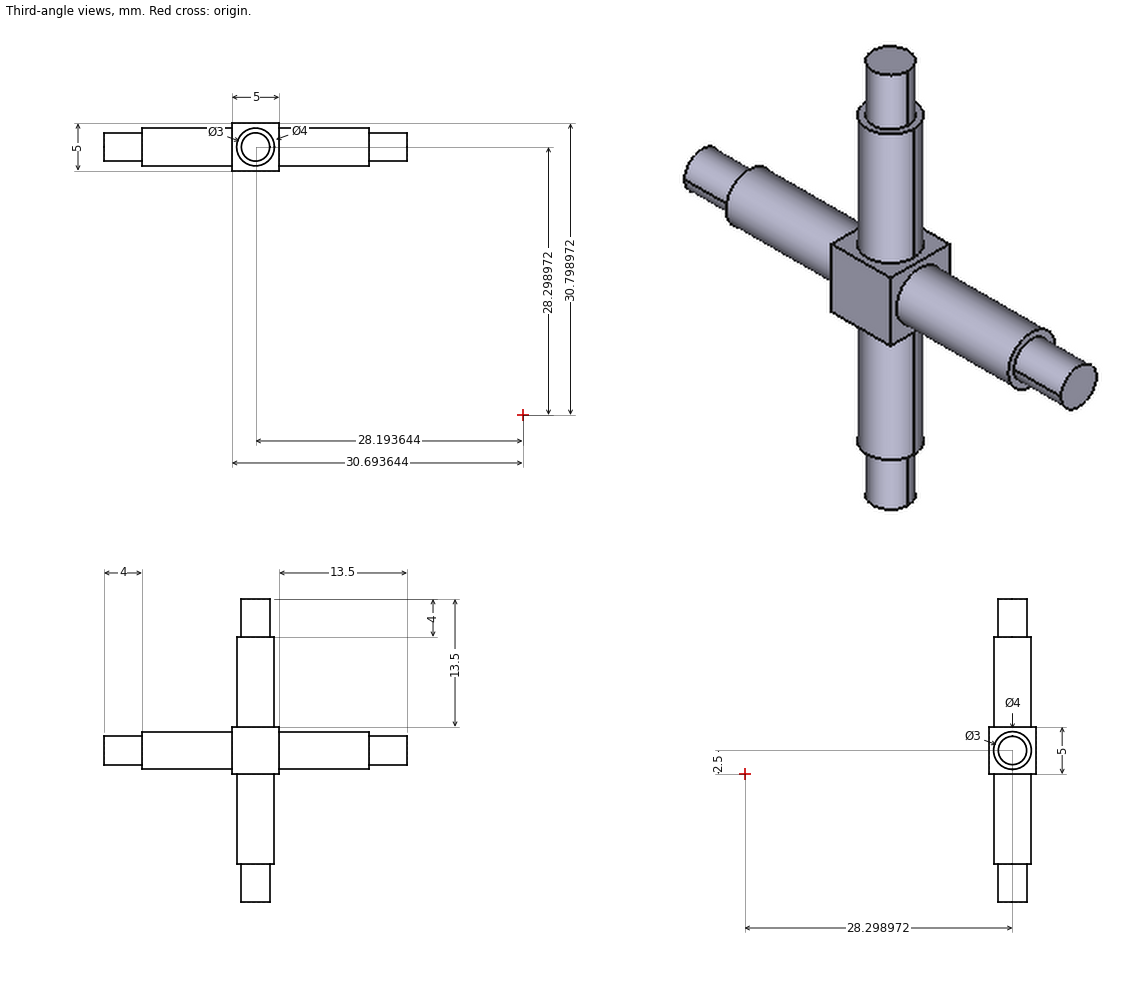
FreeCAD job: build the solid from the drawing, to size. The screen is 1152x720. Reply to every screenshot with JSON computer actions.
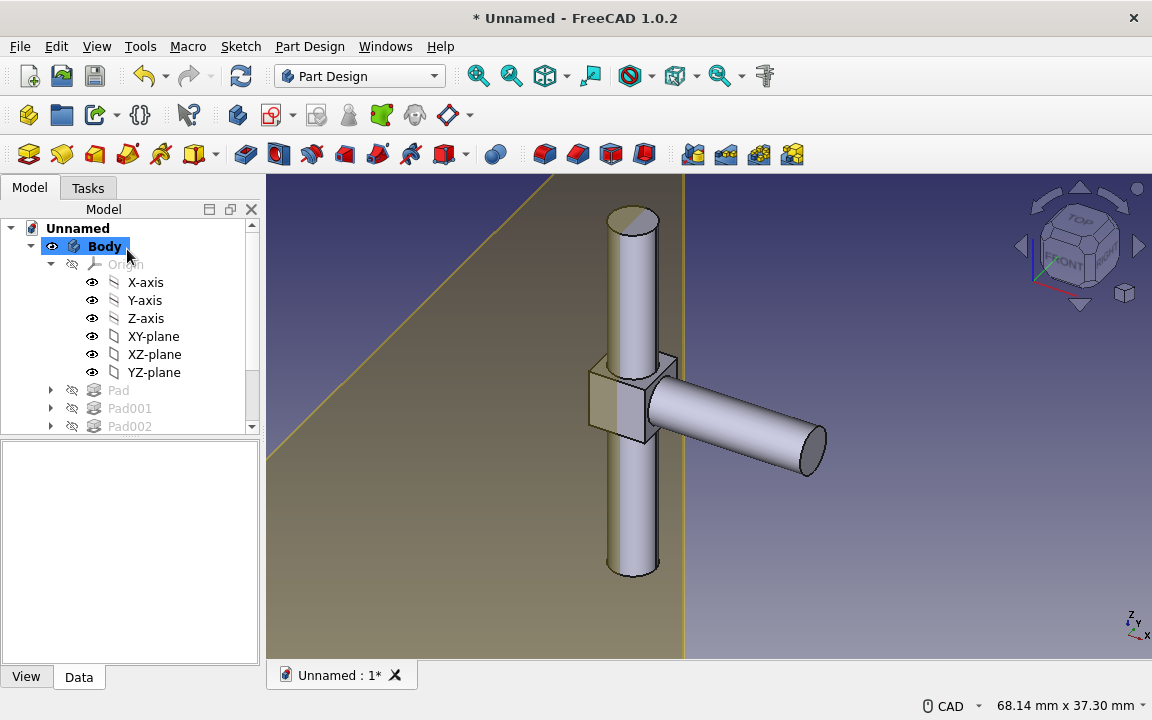
{"action": "left_click", "coordinate": [117, 426]}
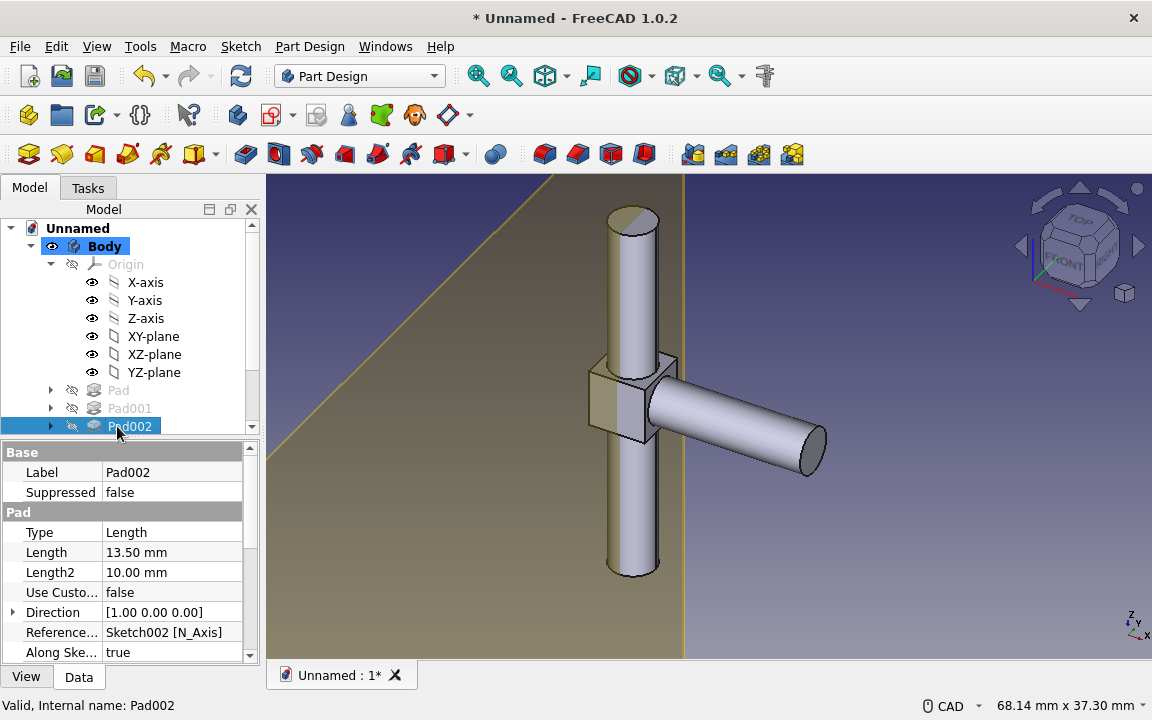
{"action": "left_click", "coordinate": [693, 154]}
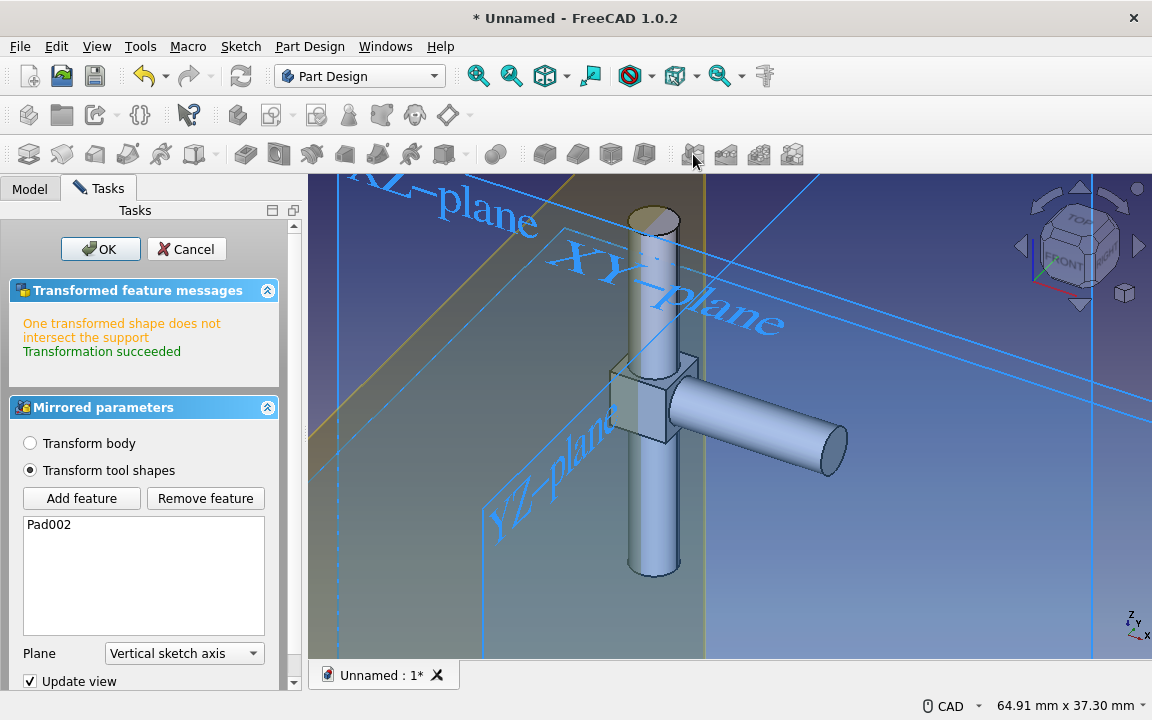
{"action": "left_click", "coordinate": [185, 654]}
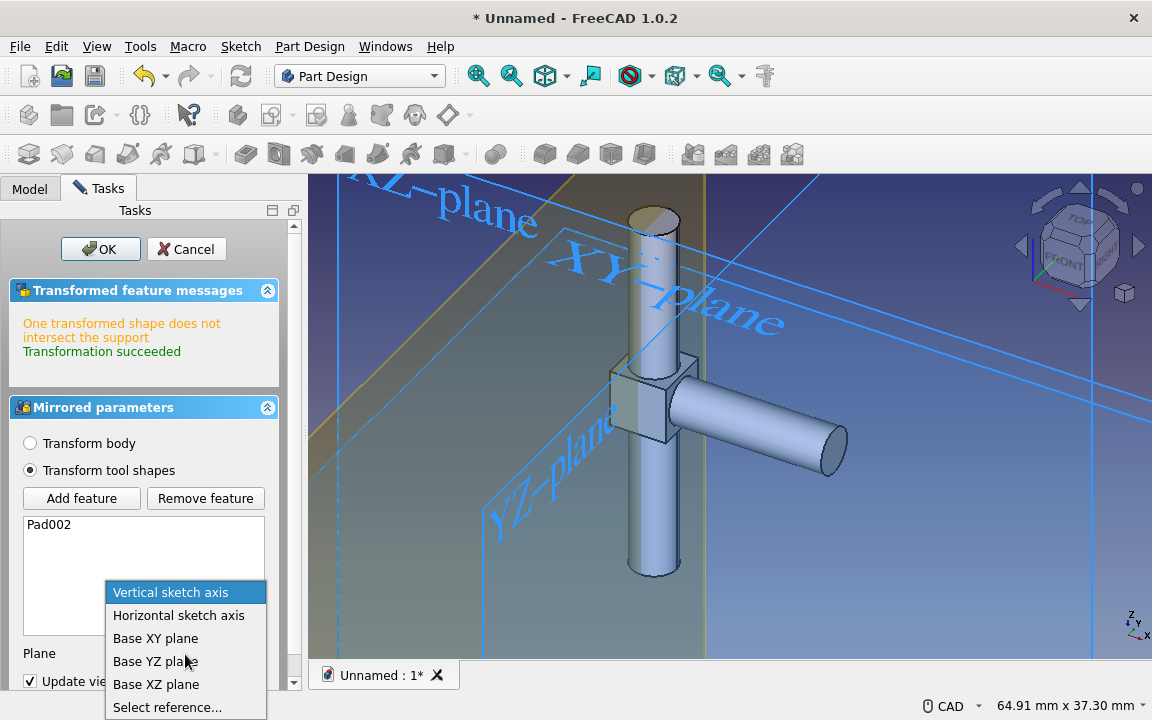
{"action": "left_click", "coordinate": [184, 708]}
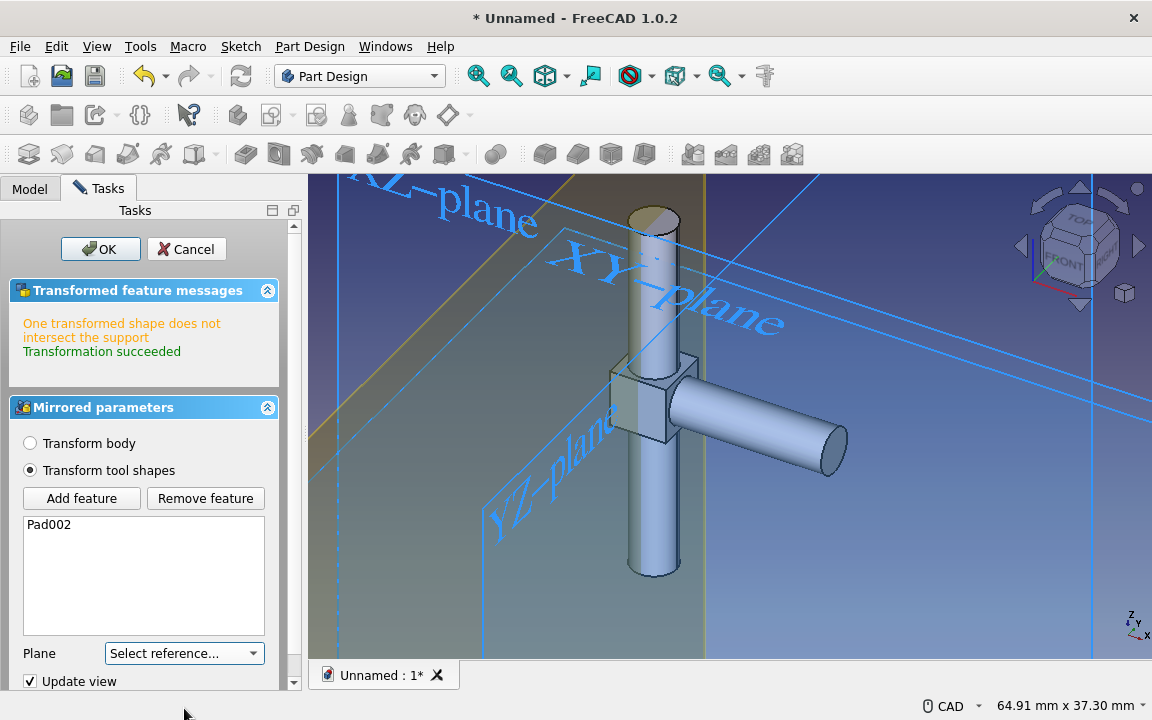
{"action": "left_click", "coordinate": [30, 188]}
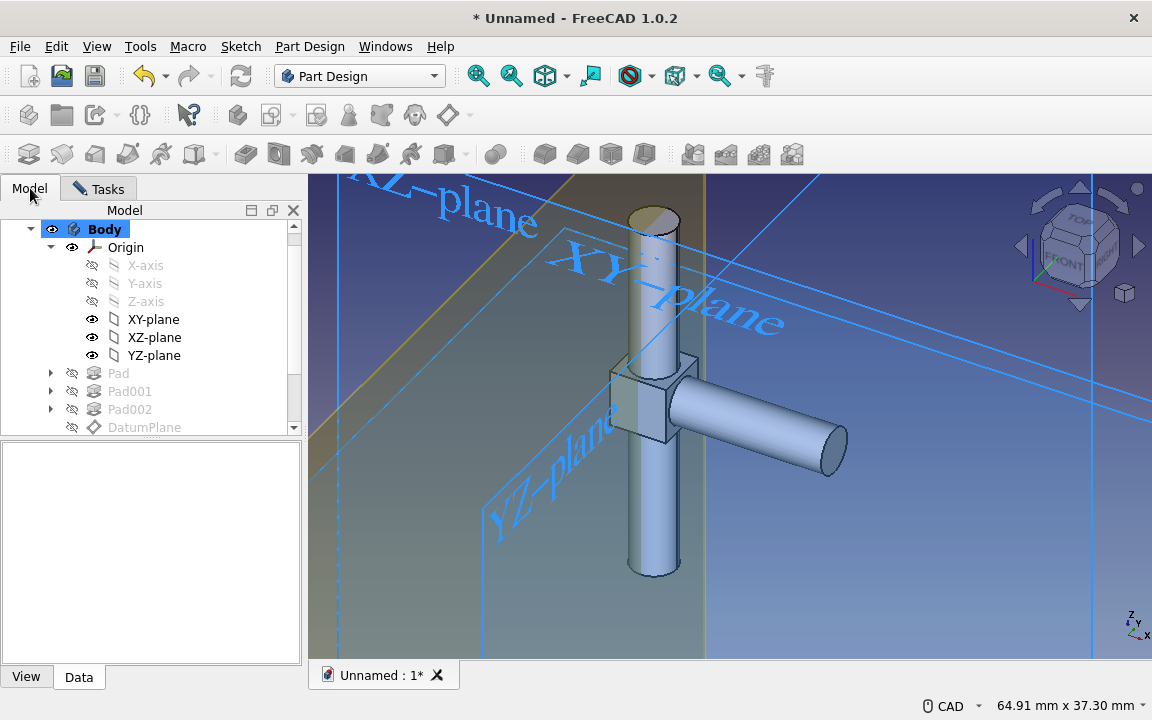
{"action": "scroll", "coordinate": [121, 333], "scroll_direction": "down", "scroll_amount": 3}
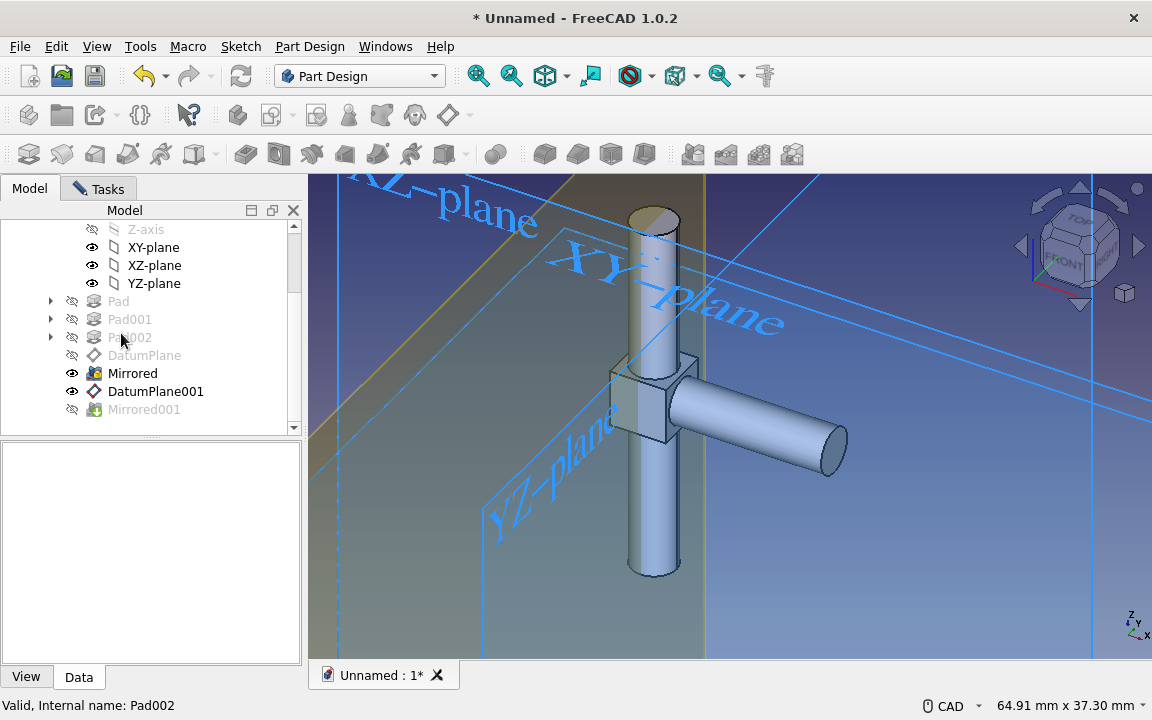
{"action": "left_click", "coordinate": [117, 391]}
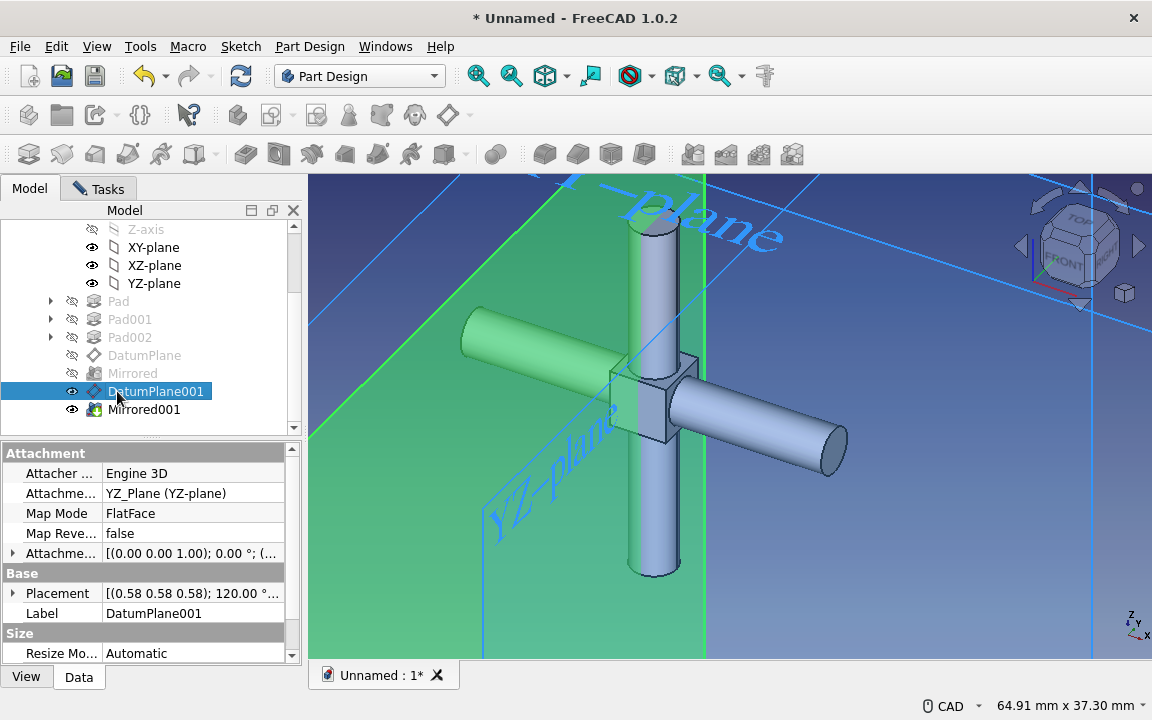
{"action": "left_click", "coordinate": [98, 188]}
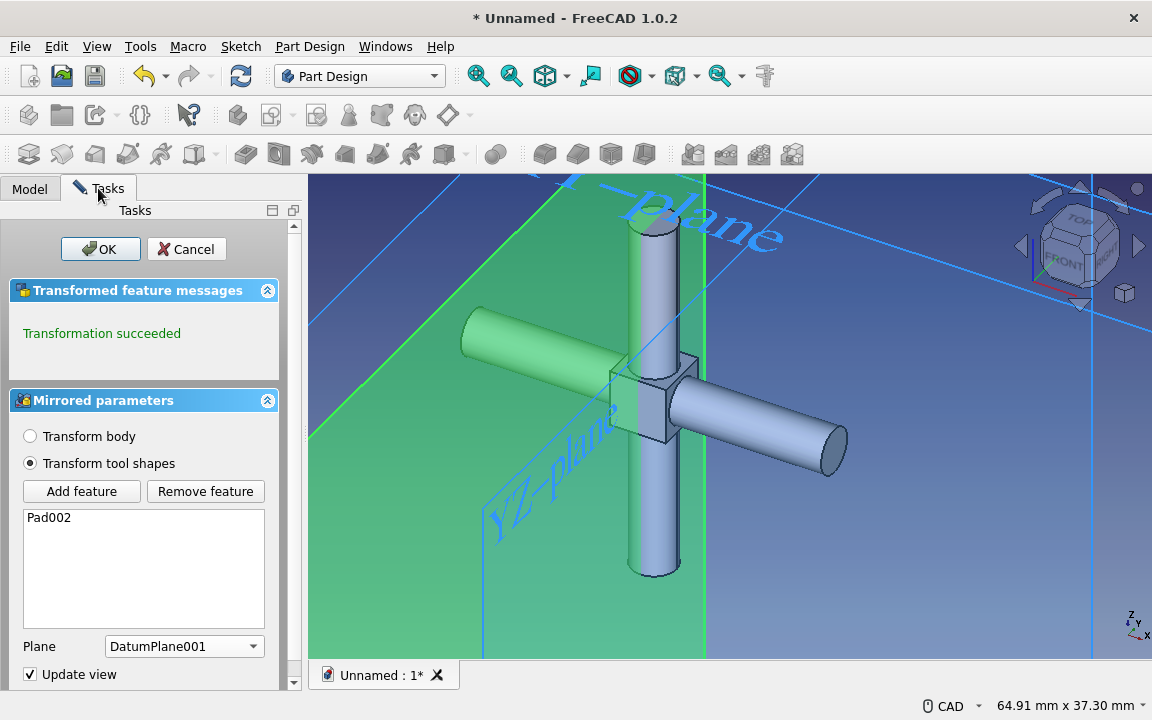
{"action": "left_click", "coordinate": [101, 249]}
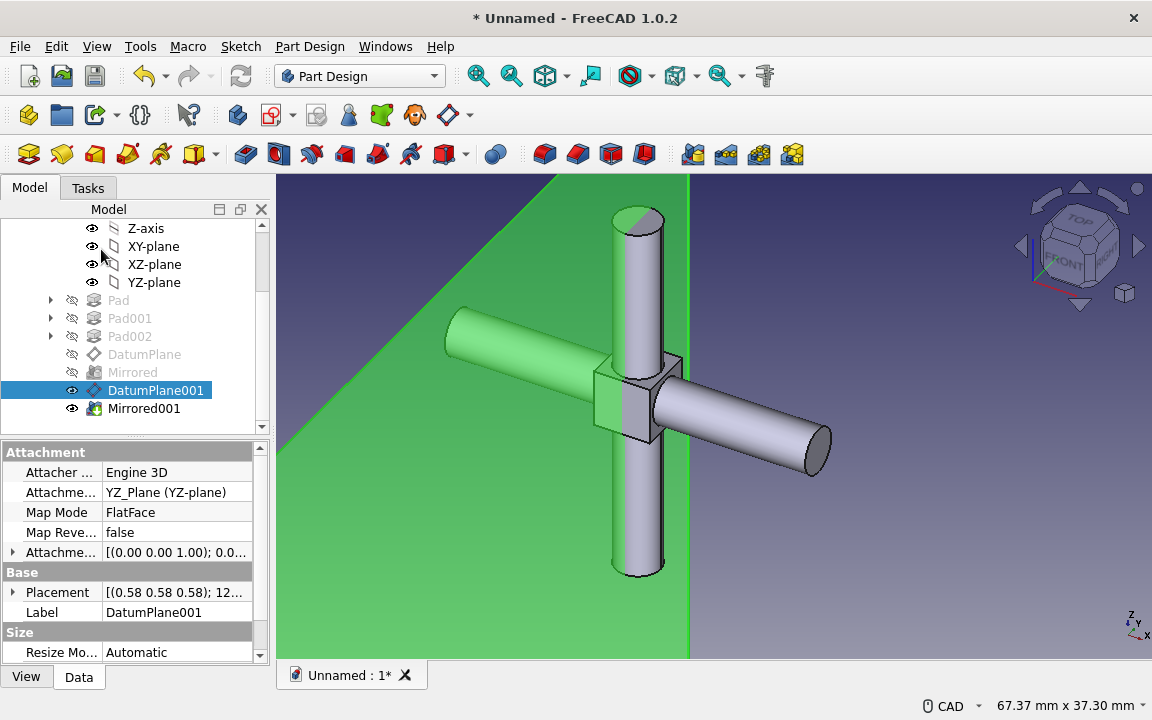
{"action": "left_click", "coordinate": [117, 390]}
{"action": "key", "text": "space"}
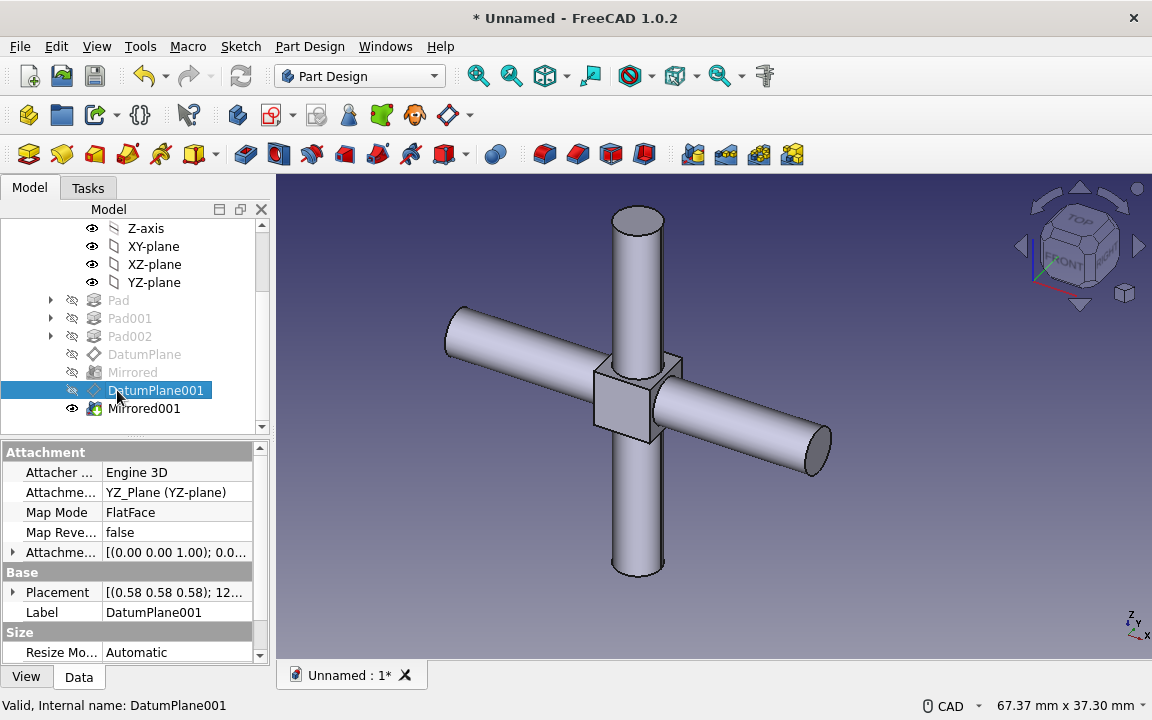
{"action": "key", "text": "v f"}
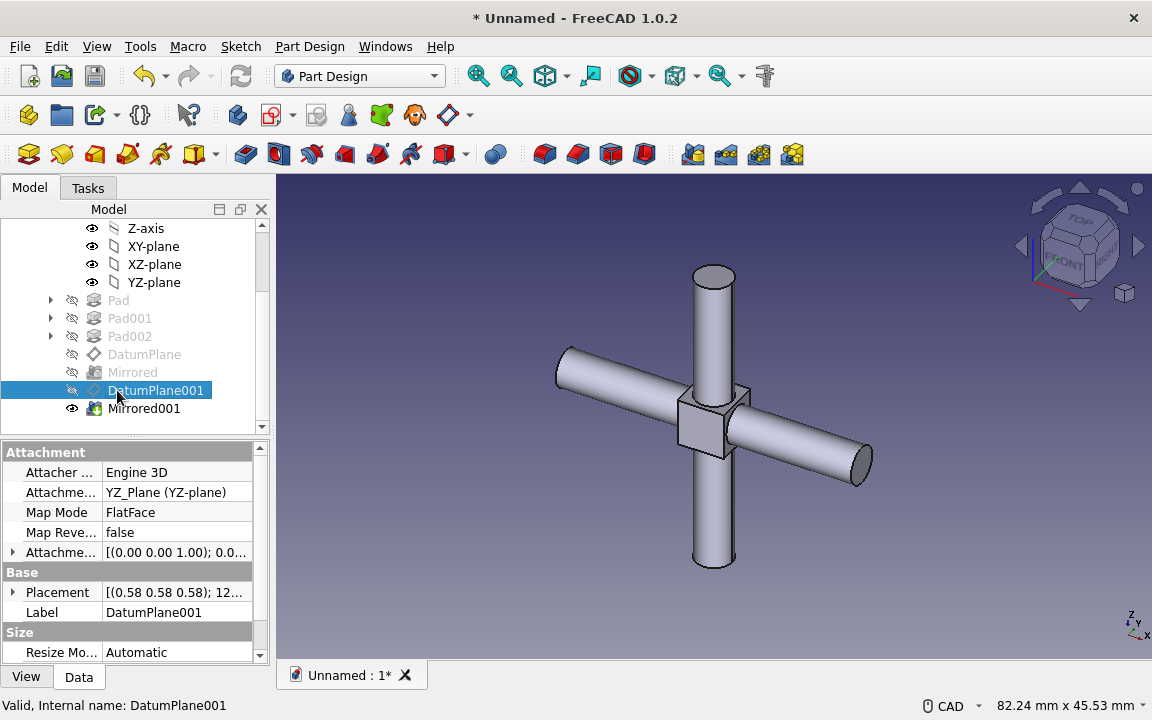
{"action": "left_click", "coordinate": [714, 276]}